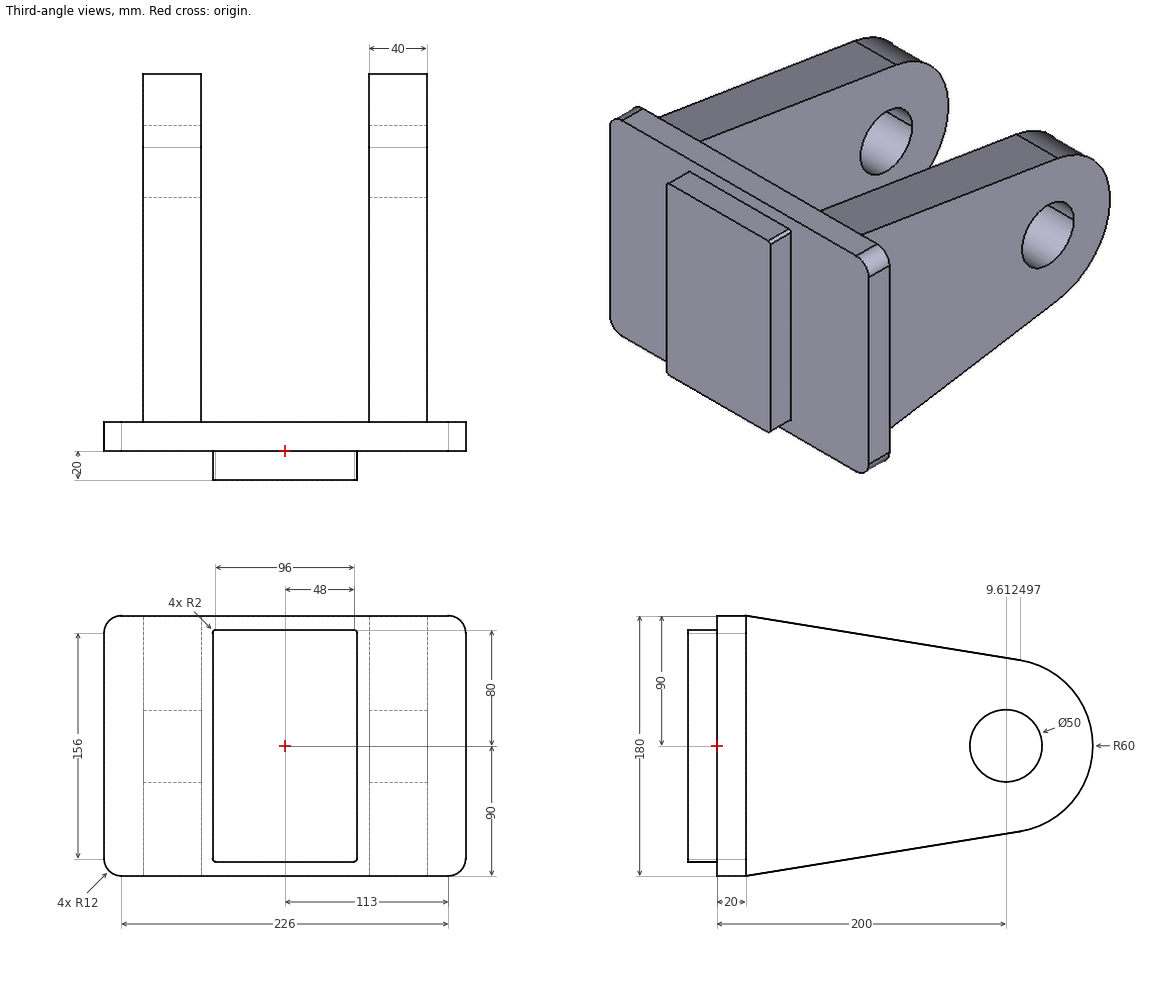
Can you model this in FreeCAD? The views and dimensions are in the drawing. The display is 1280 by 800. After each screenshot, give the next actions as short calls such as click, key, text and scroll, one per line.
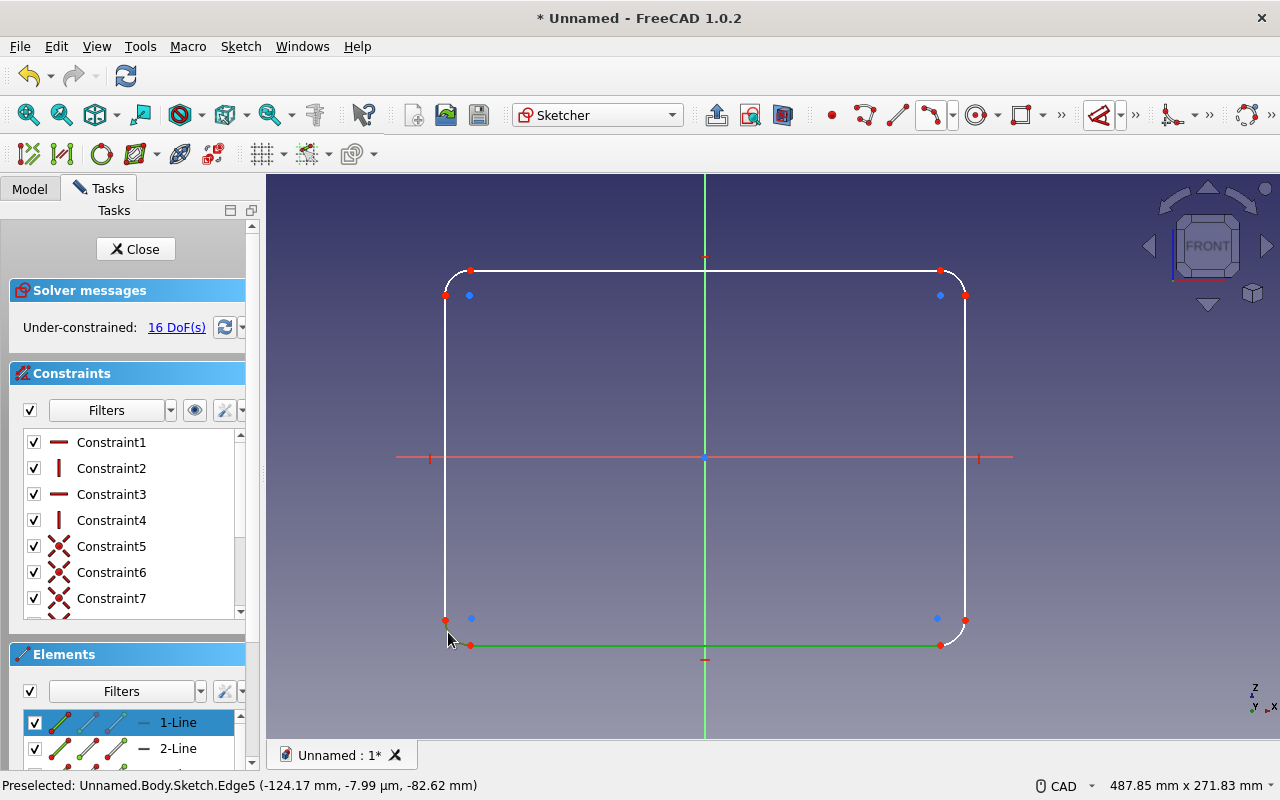
key(t)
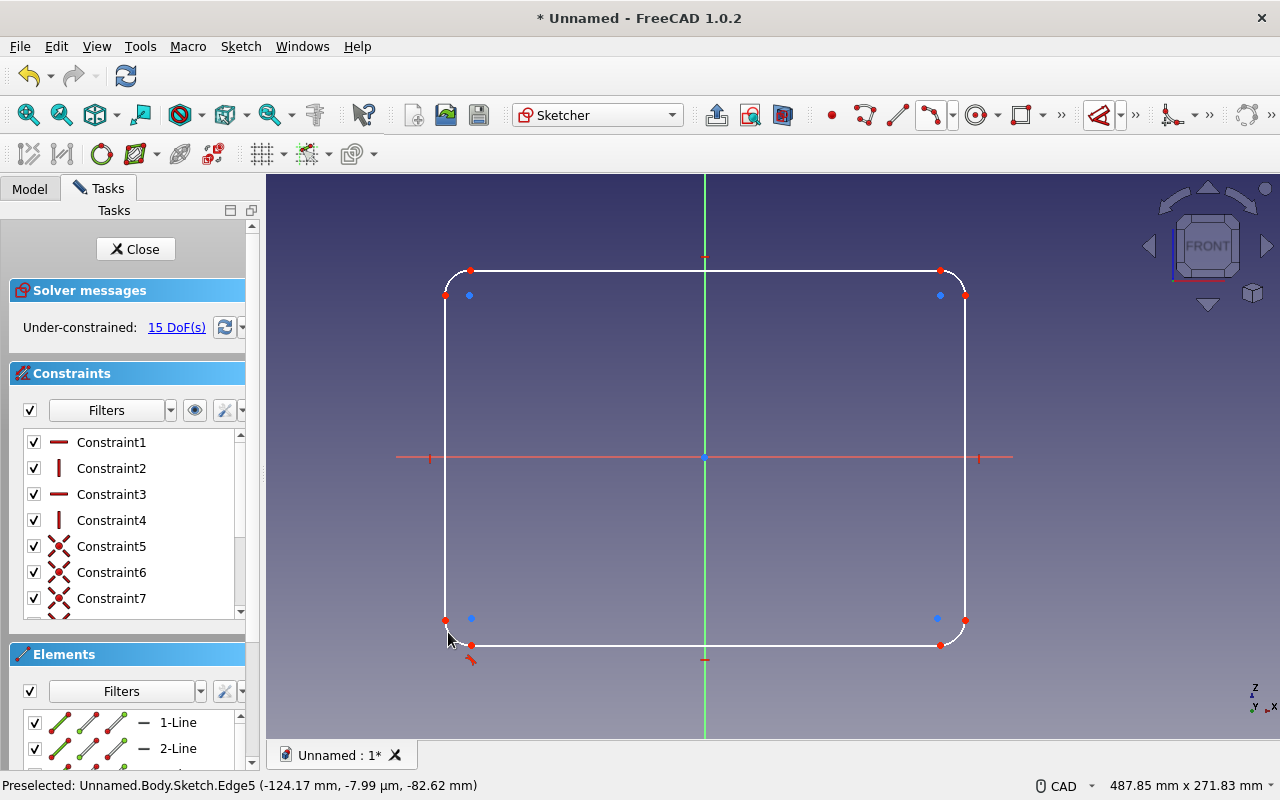
click(800, 646)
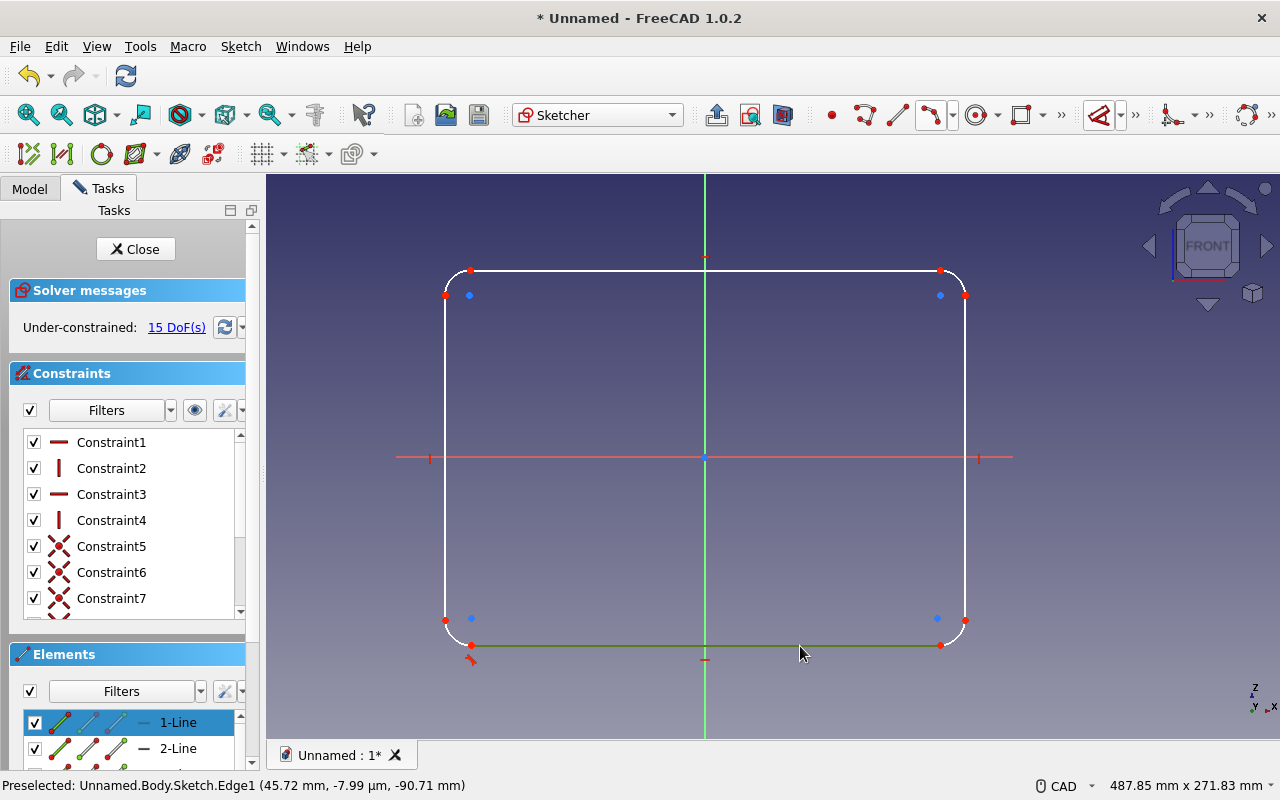
click(951, 642)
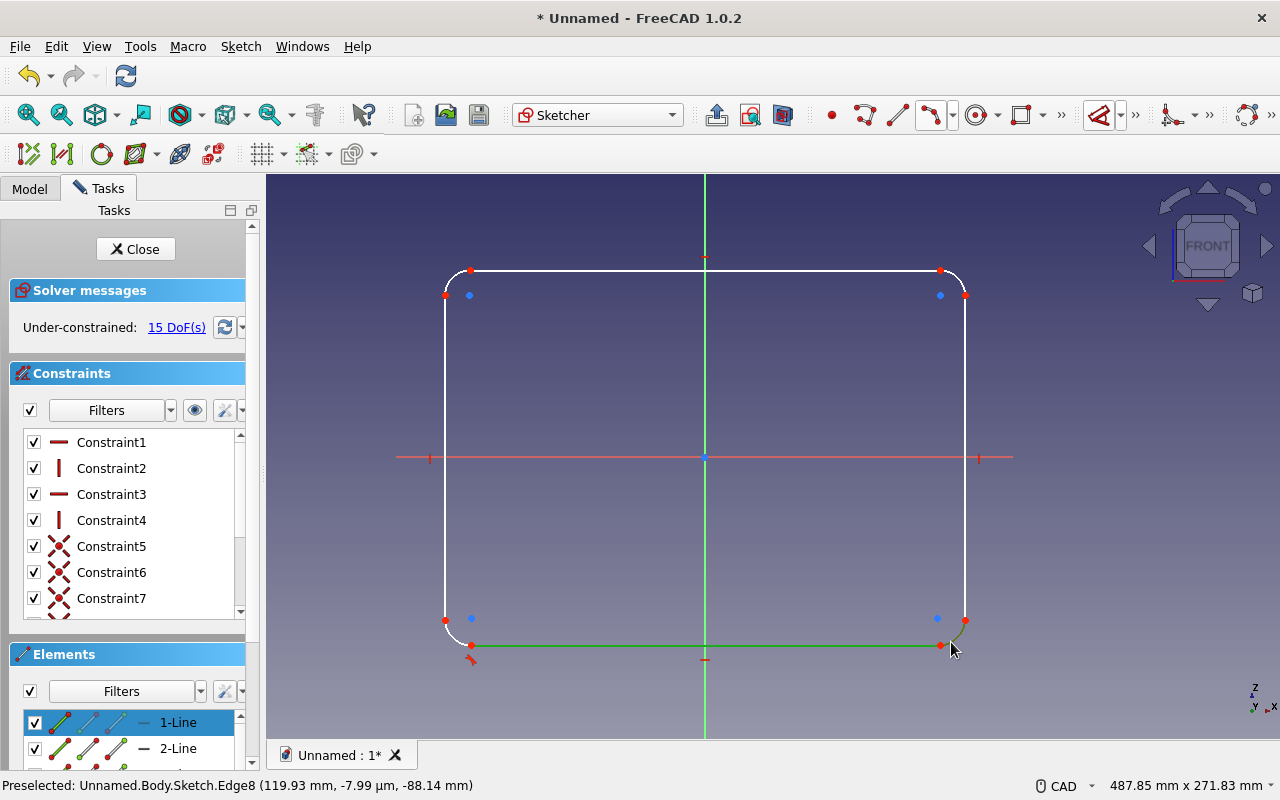
key(t)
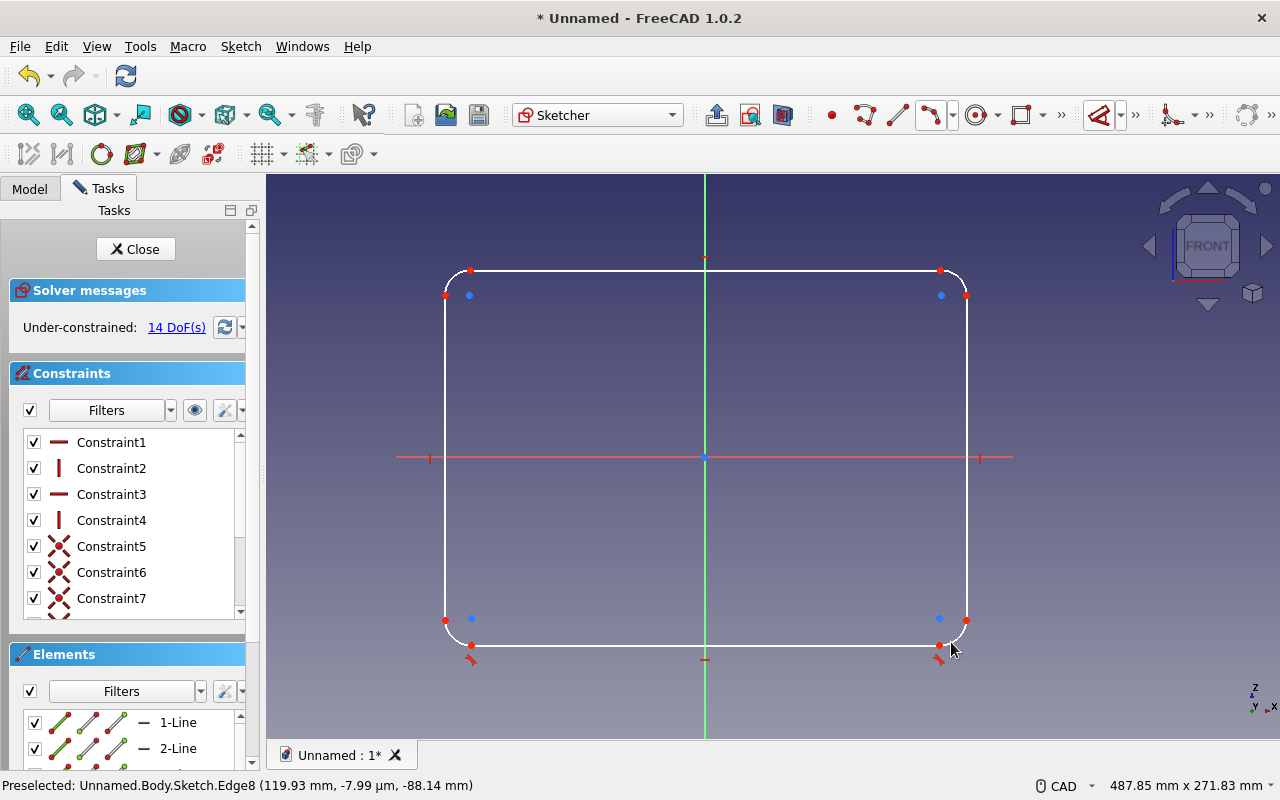
click(445, 523)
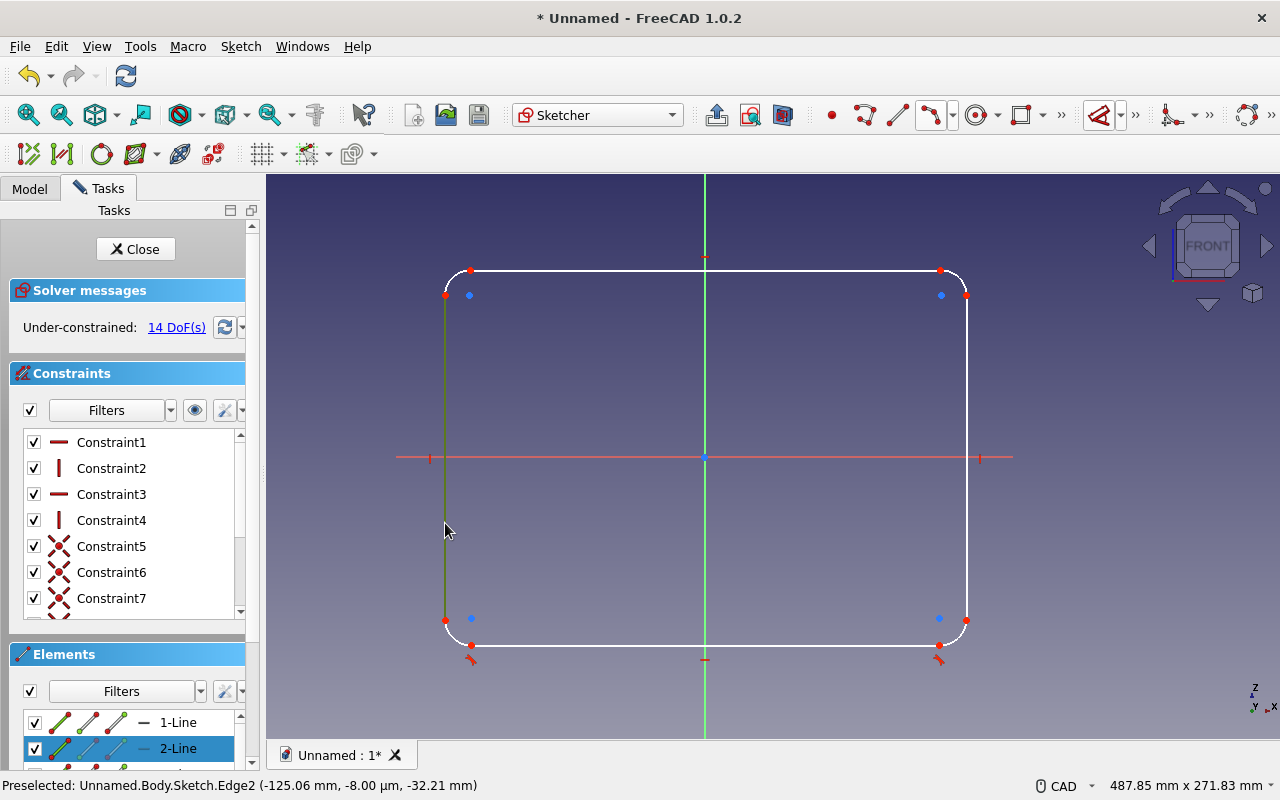
click(449, 632)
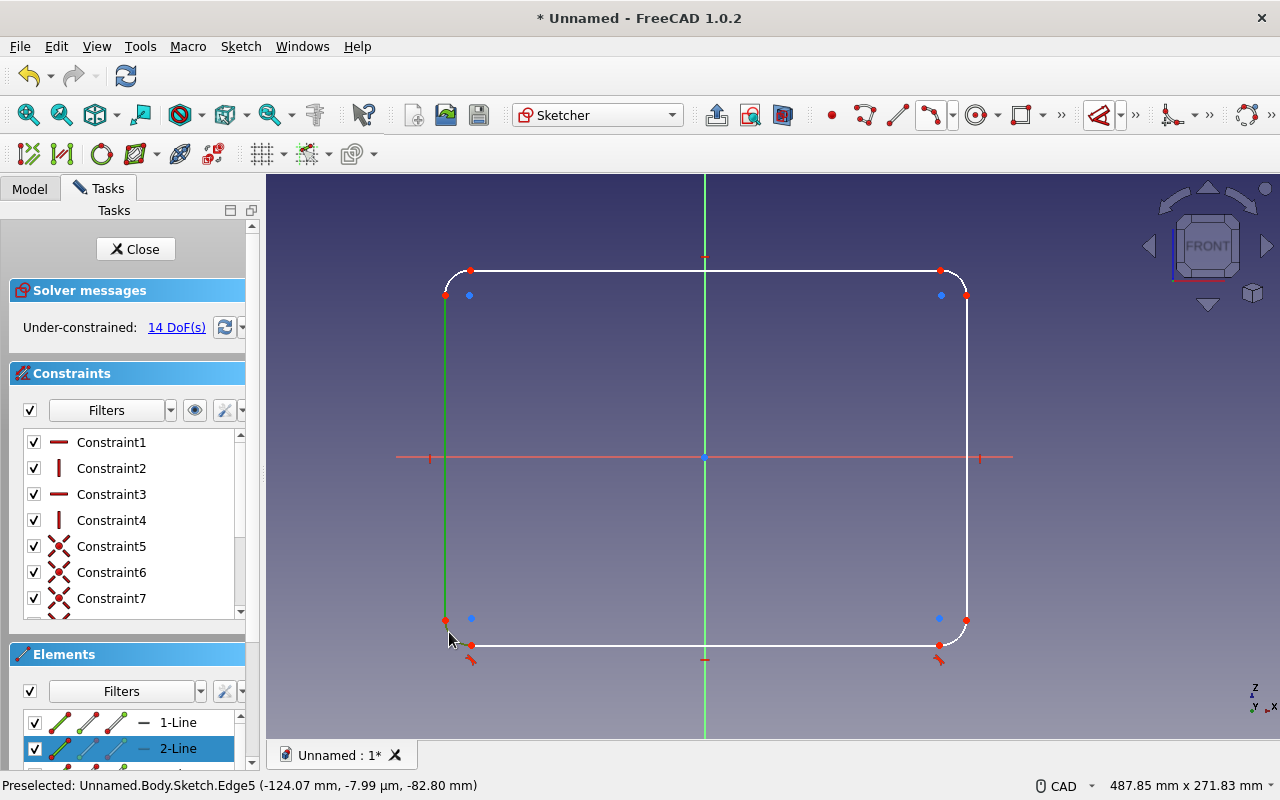
key(t)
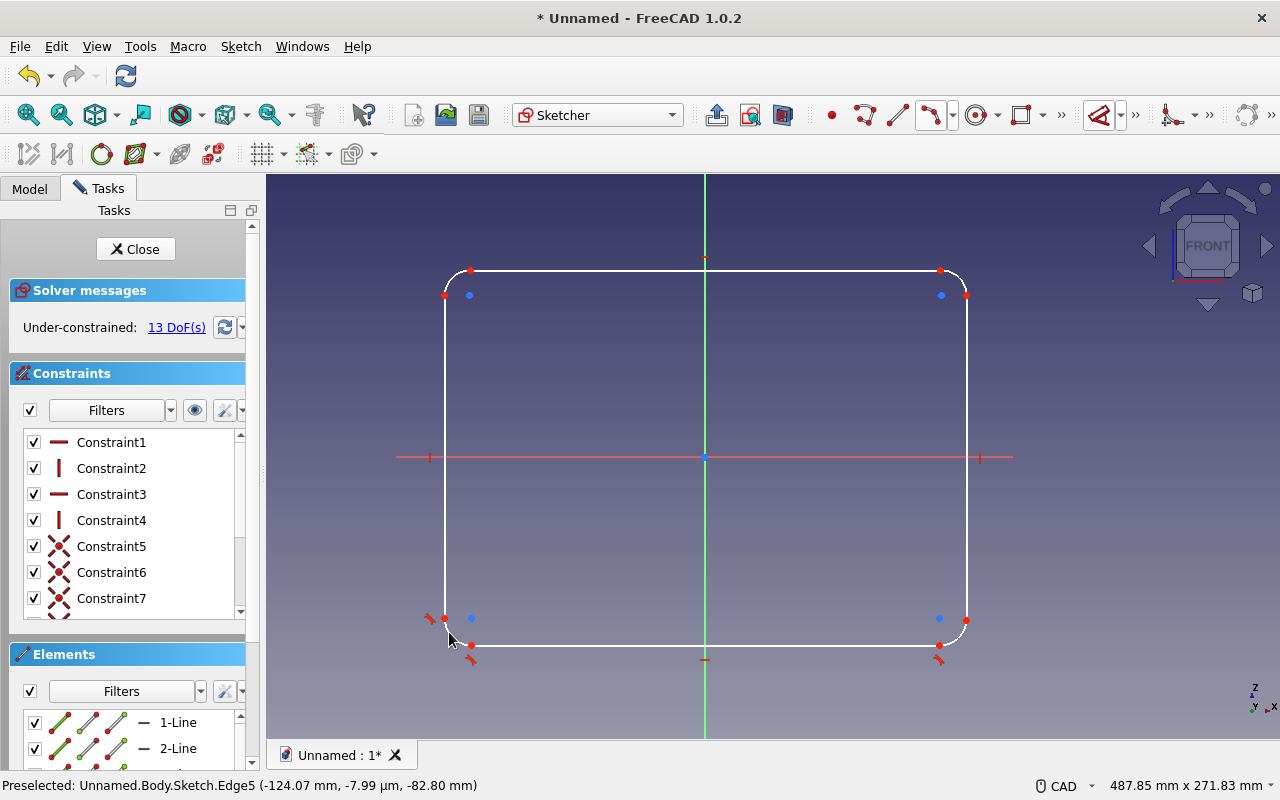
click(445, 522)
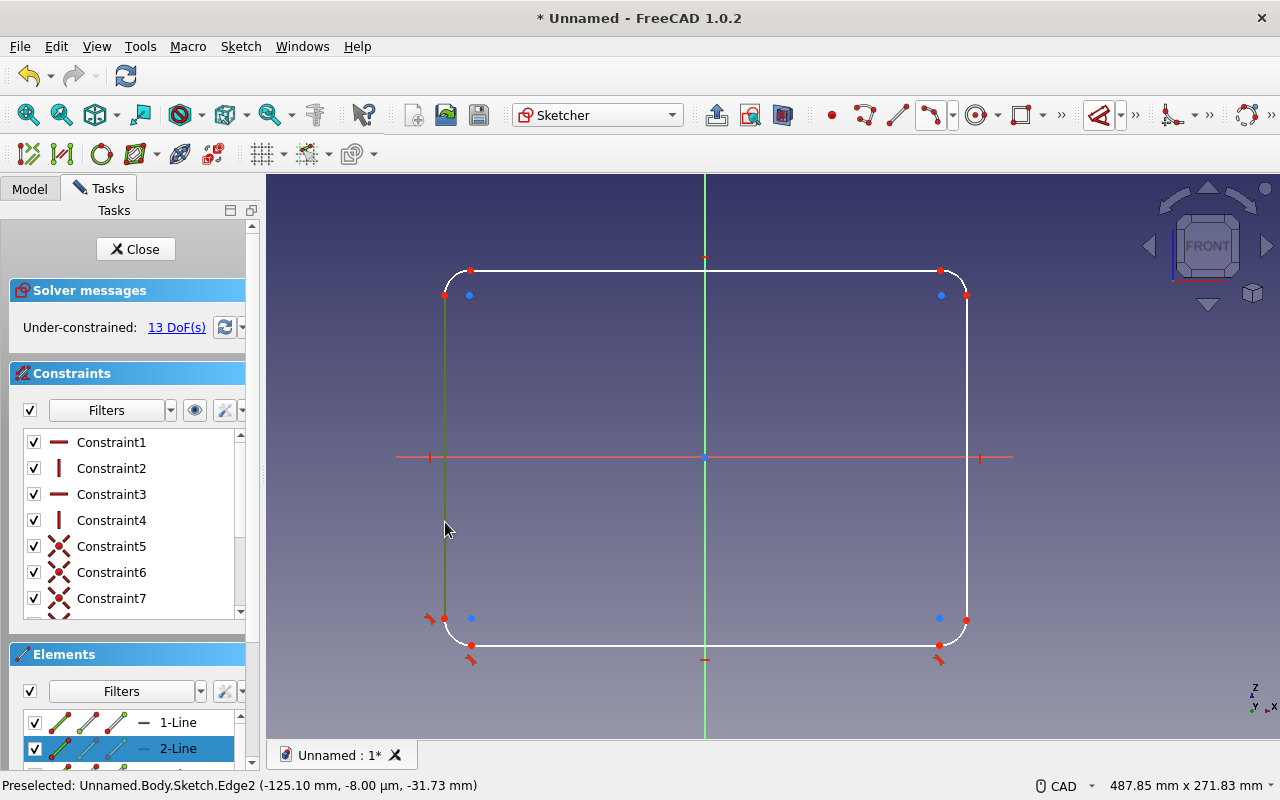
click(459, 273)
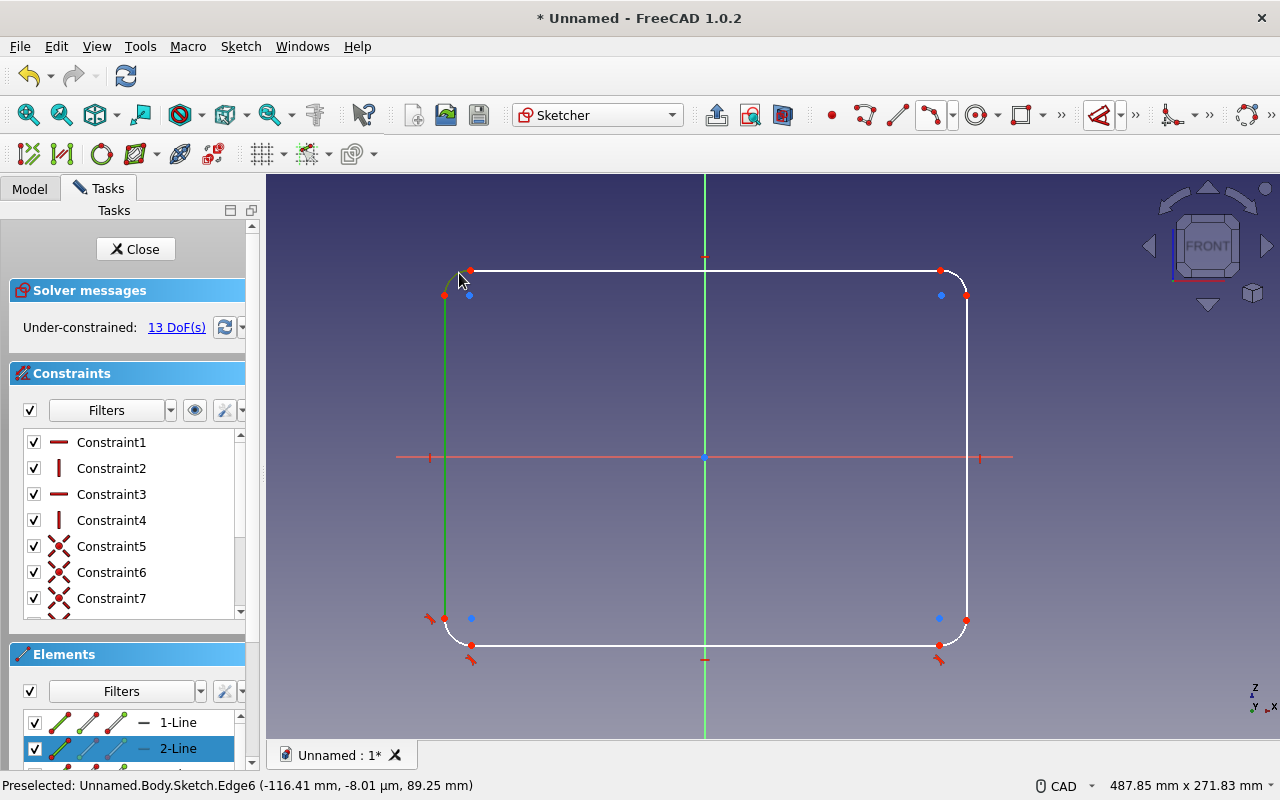
key(t)